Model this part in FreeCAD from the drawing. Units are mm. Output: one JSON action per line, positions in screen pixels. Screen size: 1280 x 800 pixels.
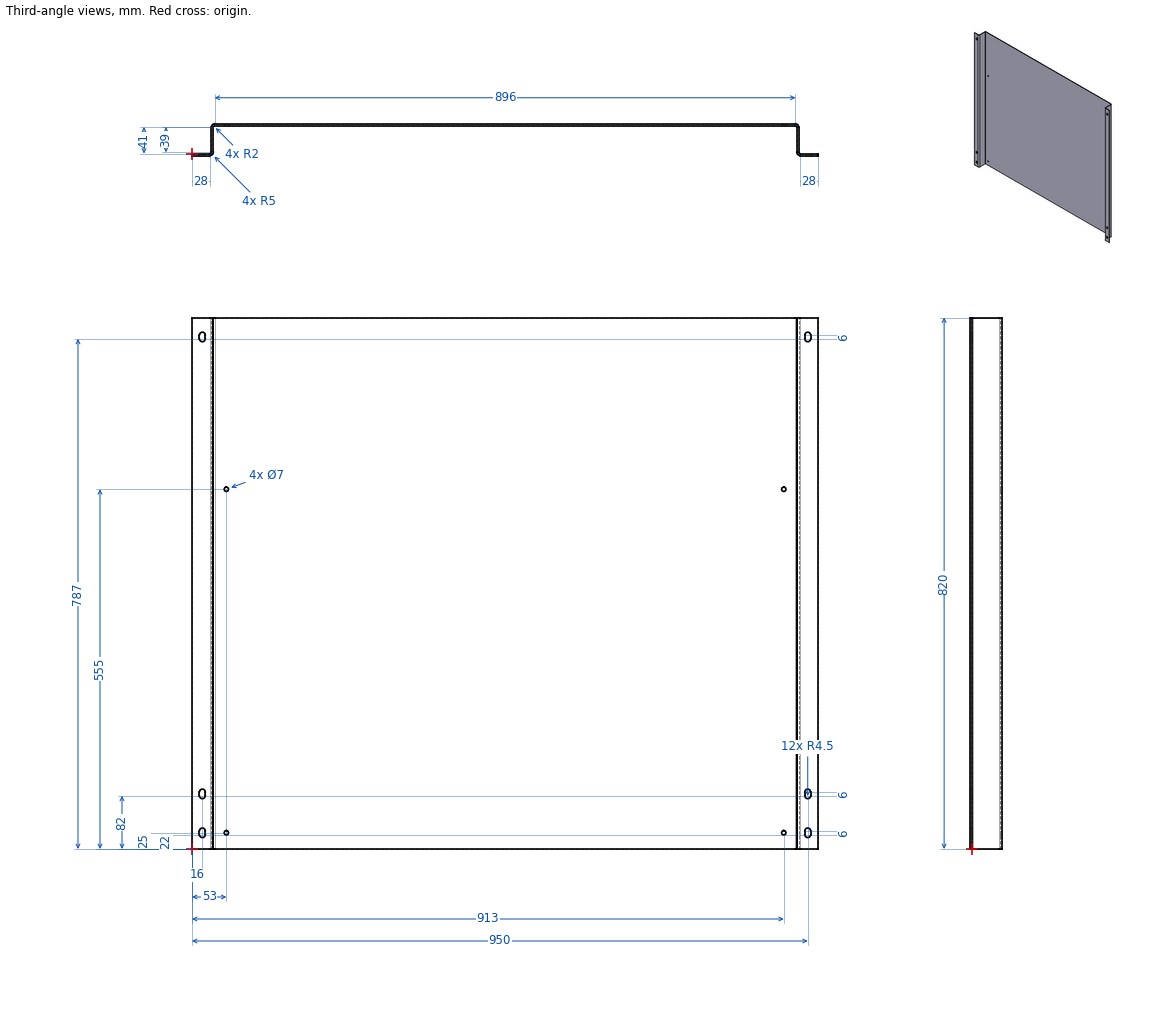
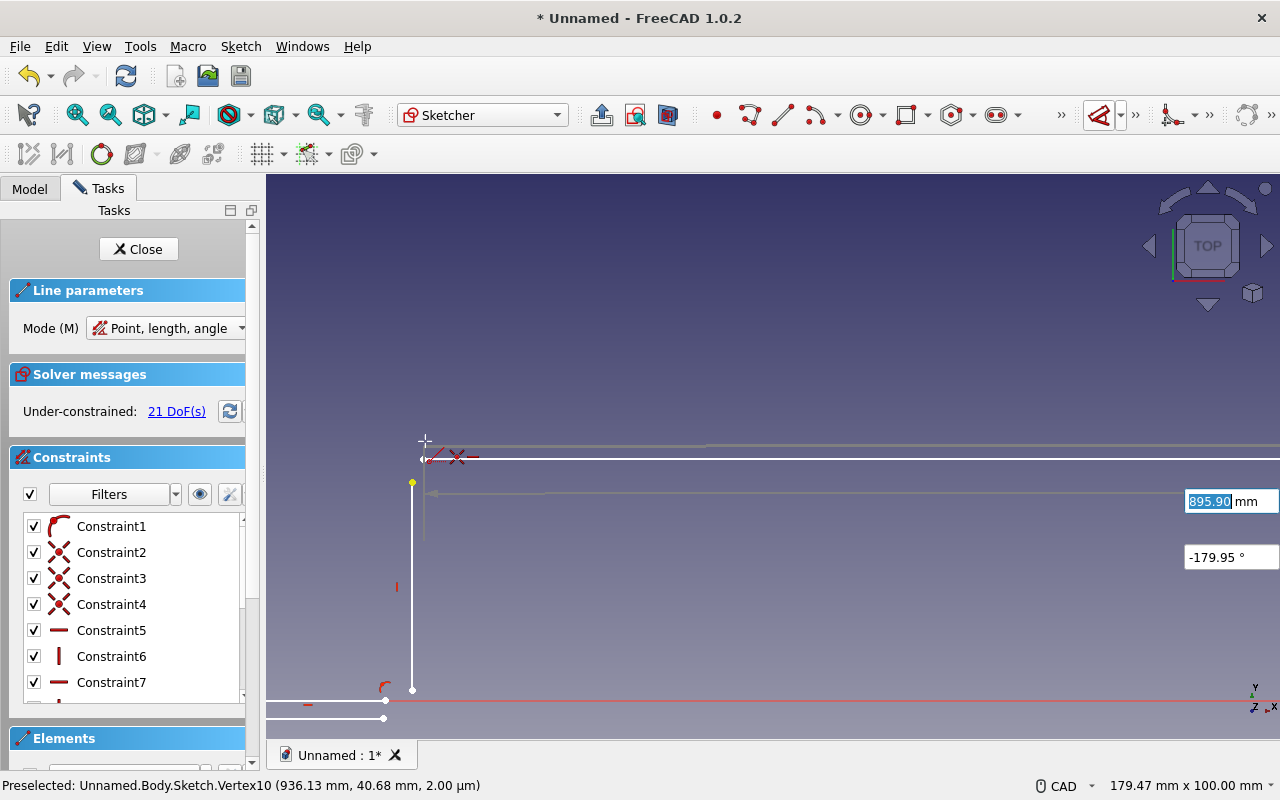
{"action": "left_click", "coordinate": [423, 441]}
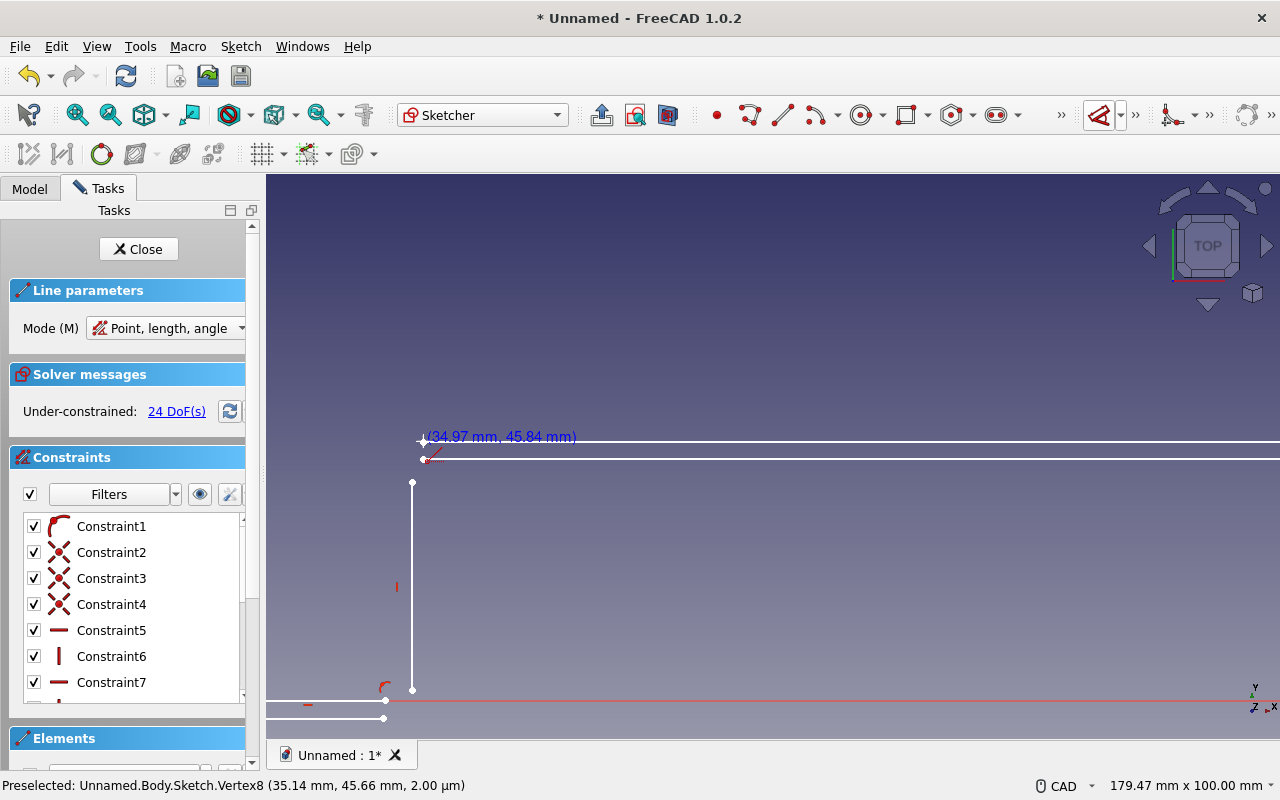
{"action": "left_click", "coordinate": [395, 469]}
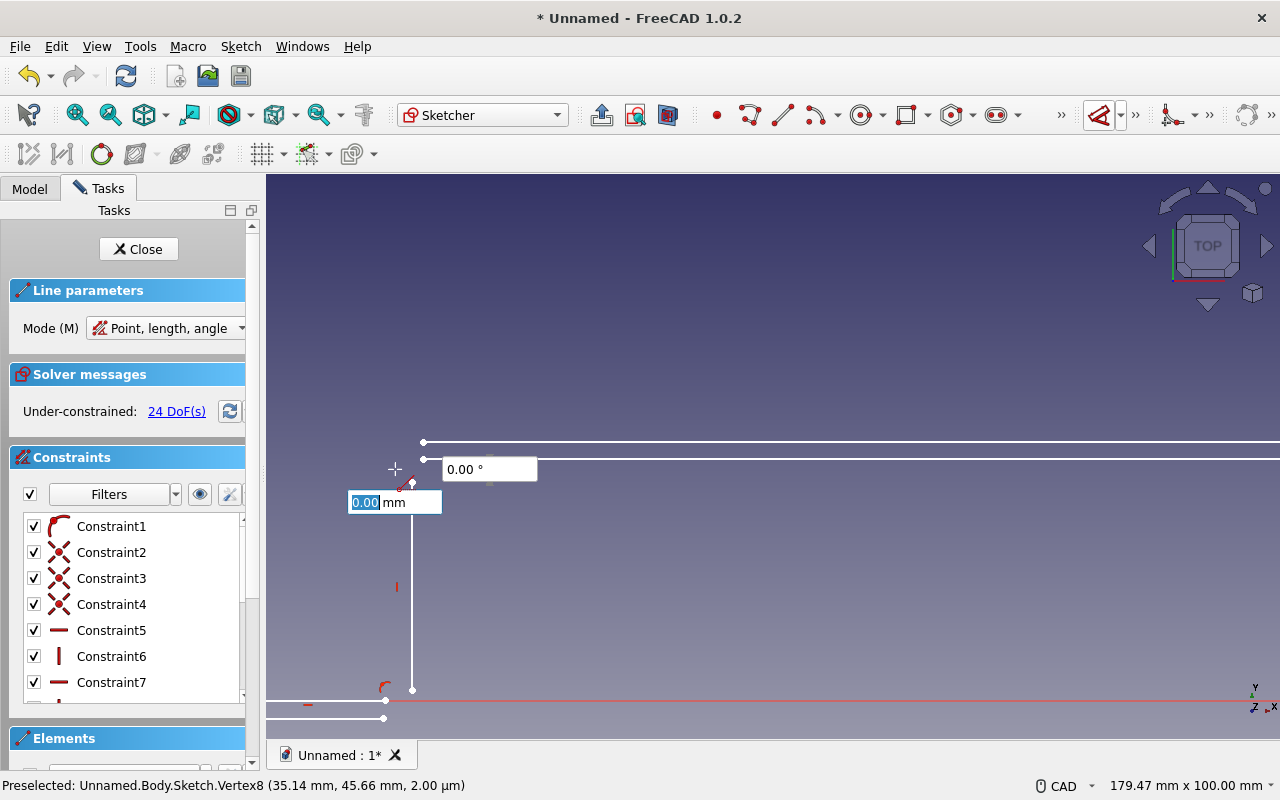
{"action": "scroll", "coordinate": [395, 690], "scroll_direction": "up", "scroll_amount": 2}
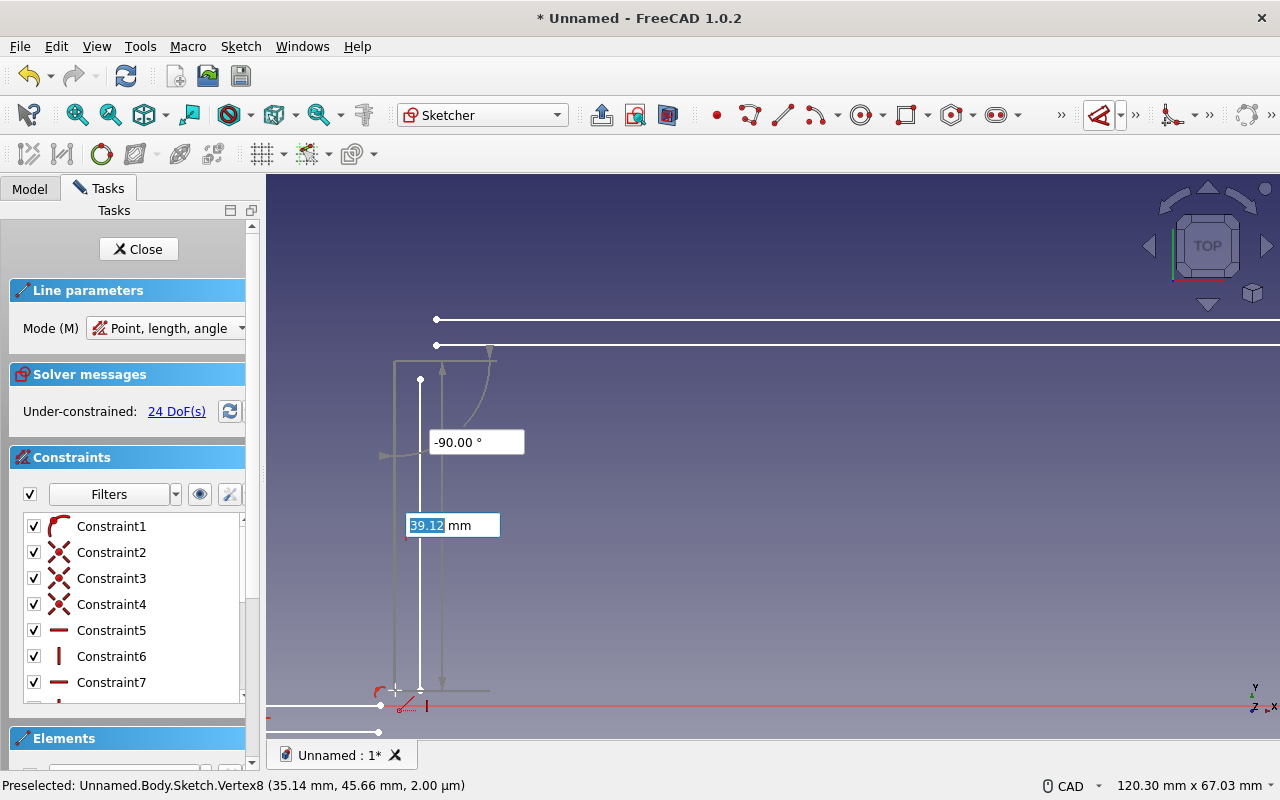
{"action": "left_click", "coordinate": [395, 689]}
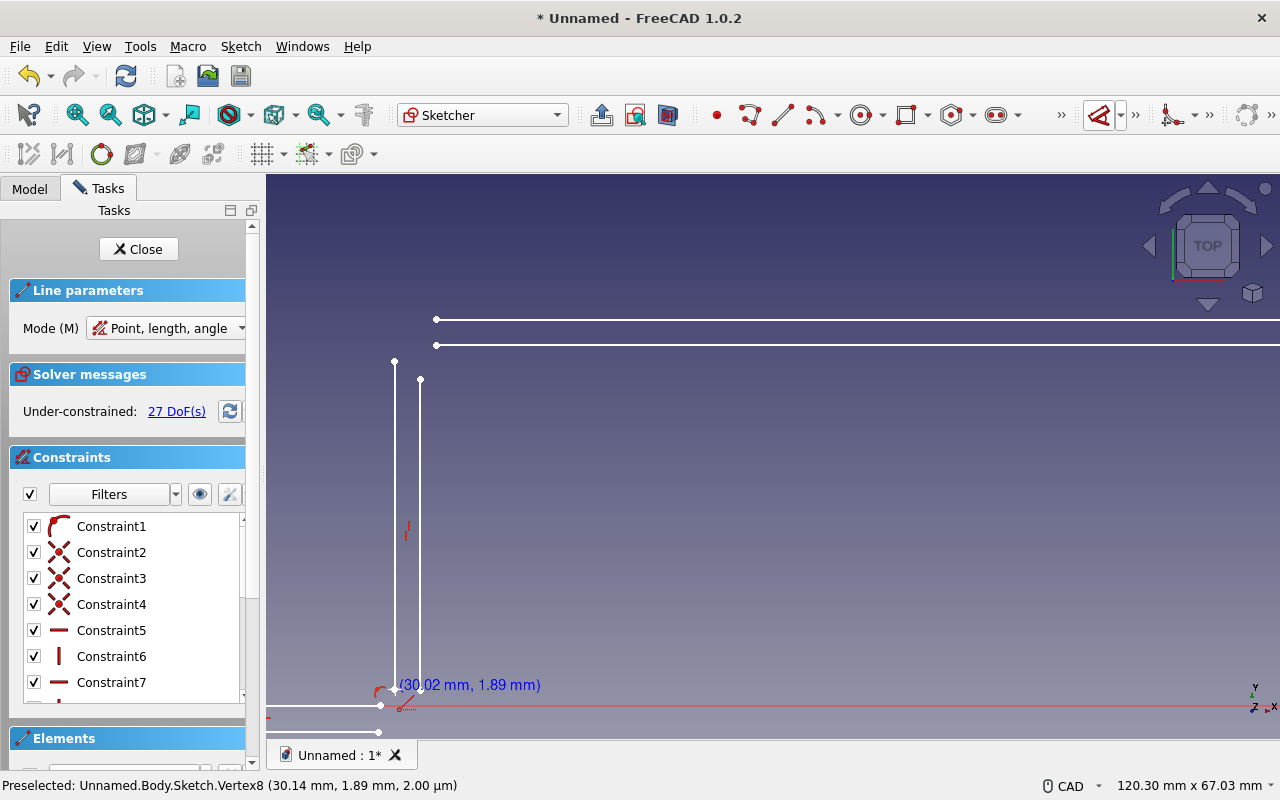
{"action": "key", "text": "g 3 a"}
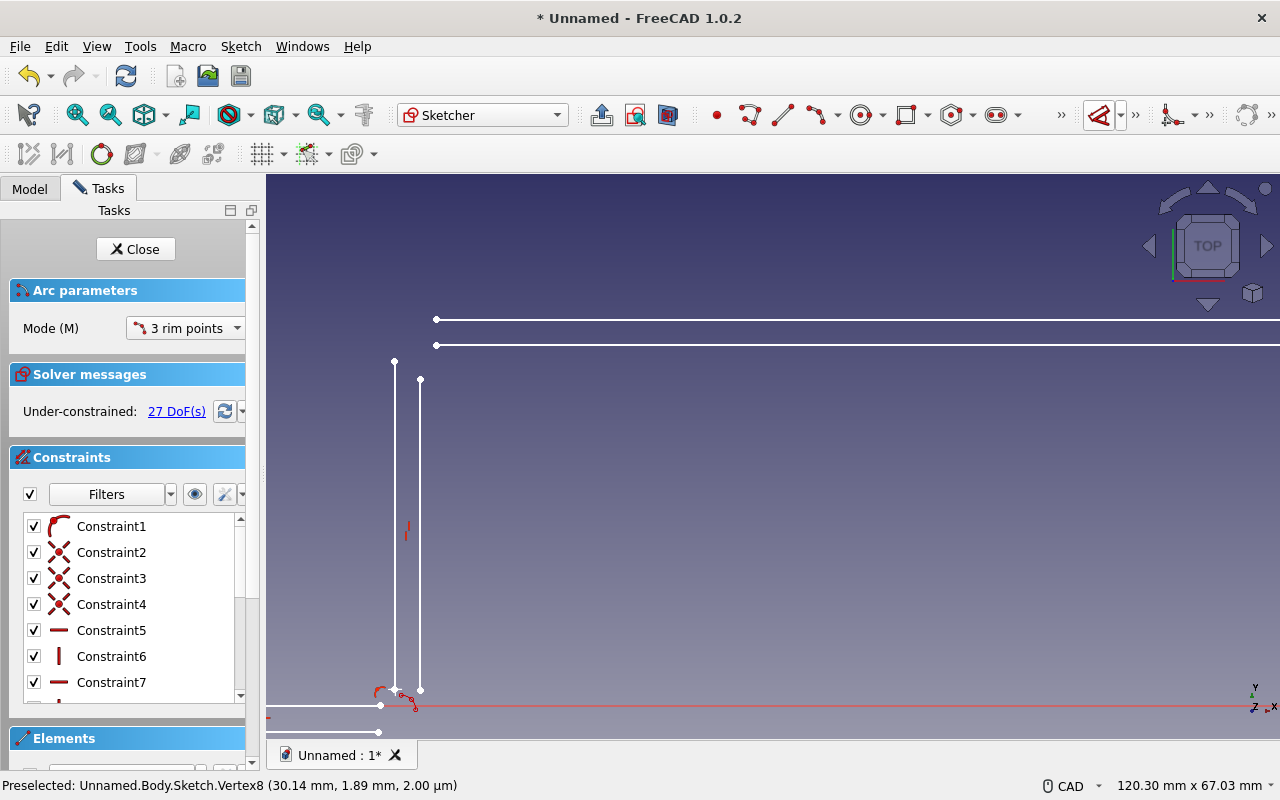
{"action": "scroll", "coordinate": [423, 451], "scroll_direction": "down", "scroll_amount": 13}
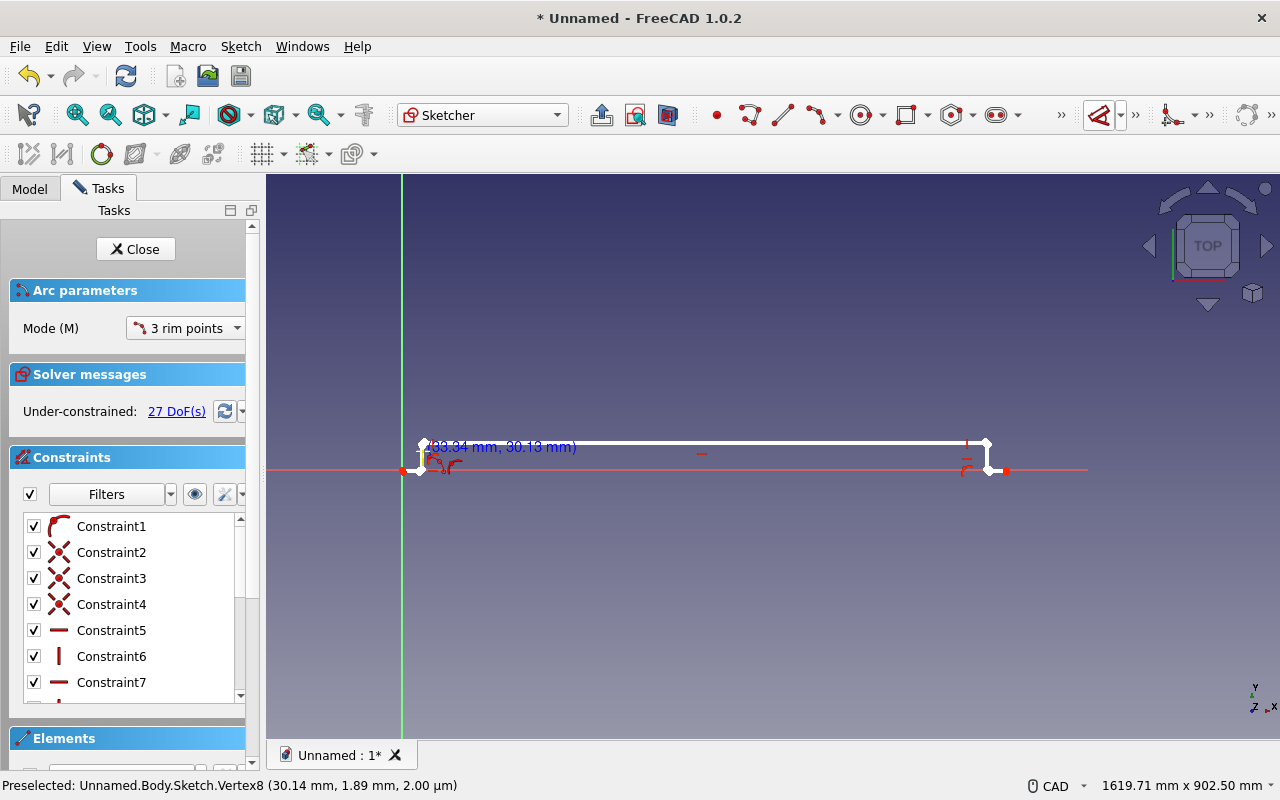
{"action": "scroll", "coordinate": [420, 472], "scroll_direction": "up", "scroll_amount": 11}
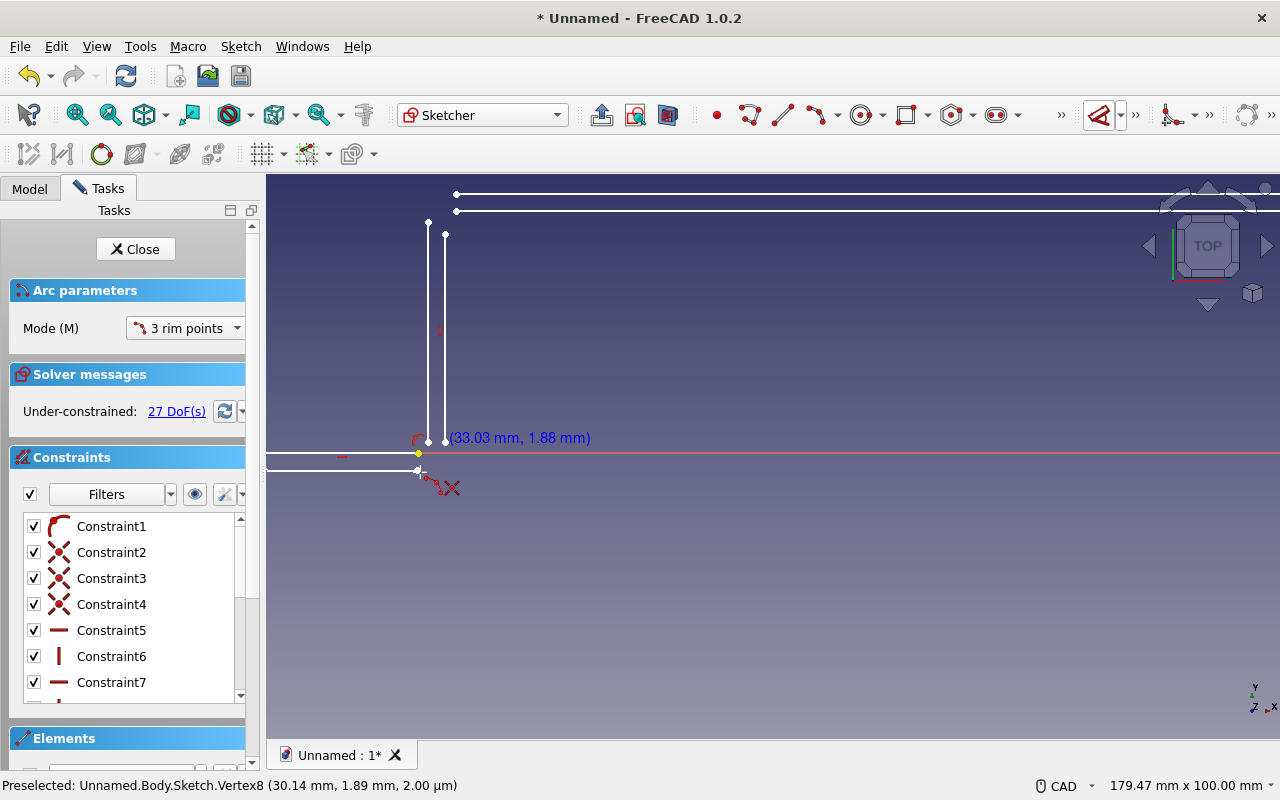
{"action": "left_click", "coordinate": [417, 471]}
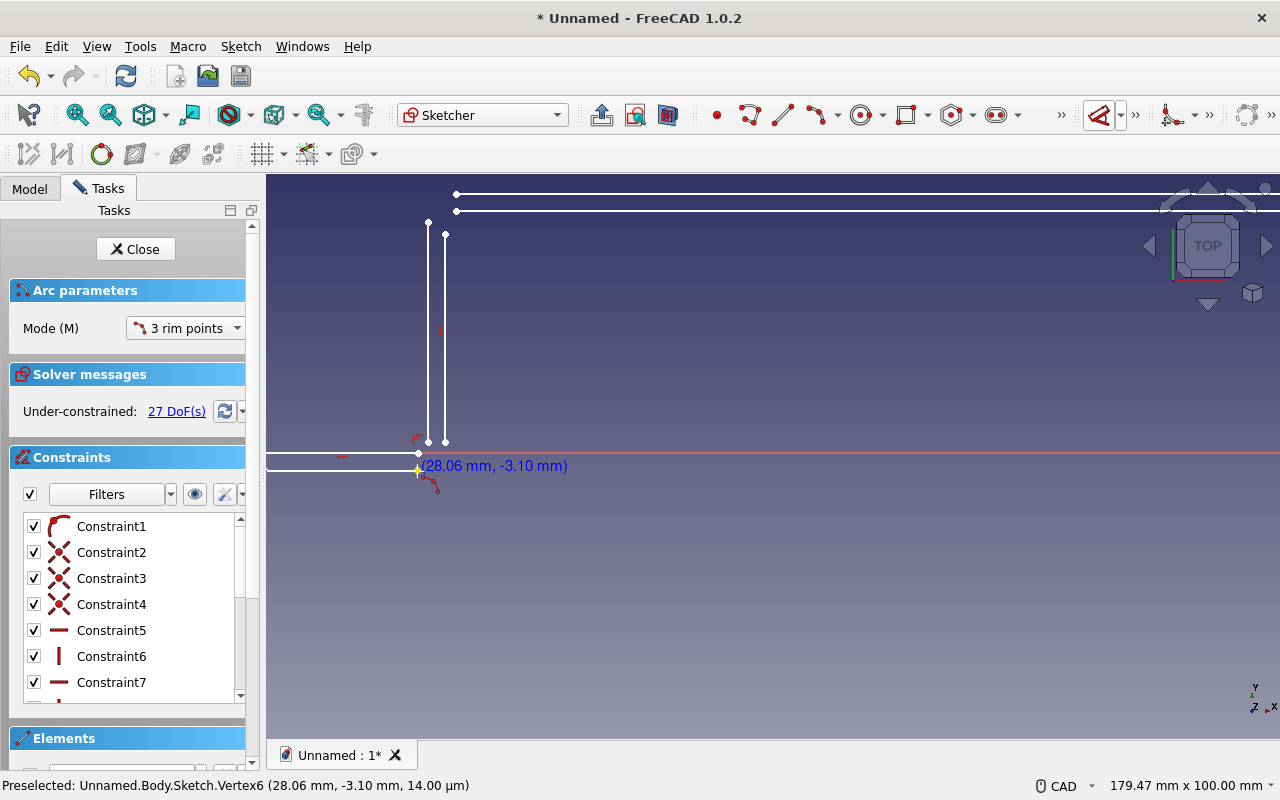
{"action": "scroll", "coordinate": [445, 442], "scroll_direction": "up", "scroll_amount": 2}